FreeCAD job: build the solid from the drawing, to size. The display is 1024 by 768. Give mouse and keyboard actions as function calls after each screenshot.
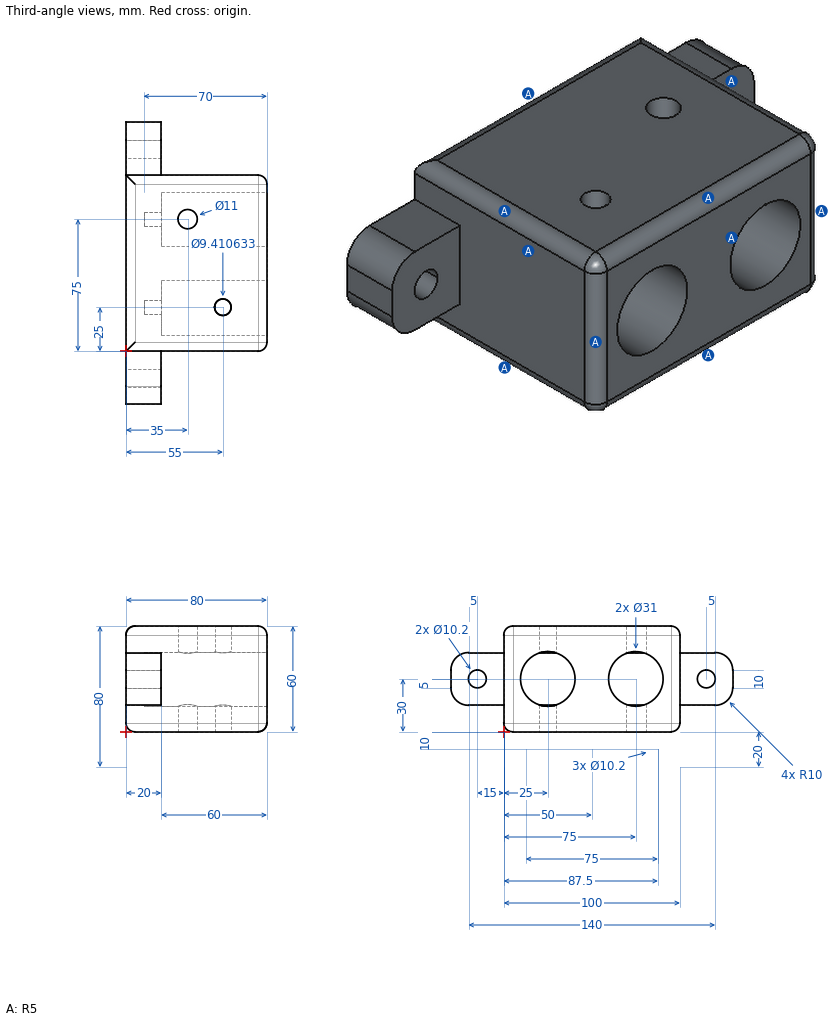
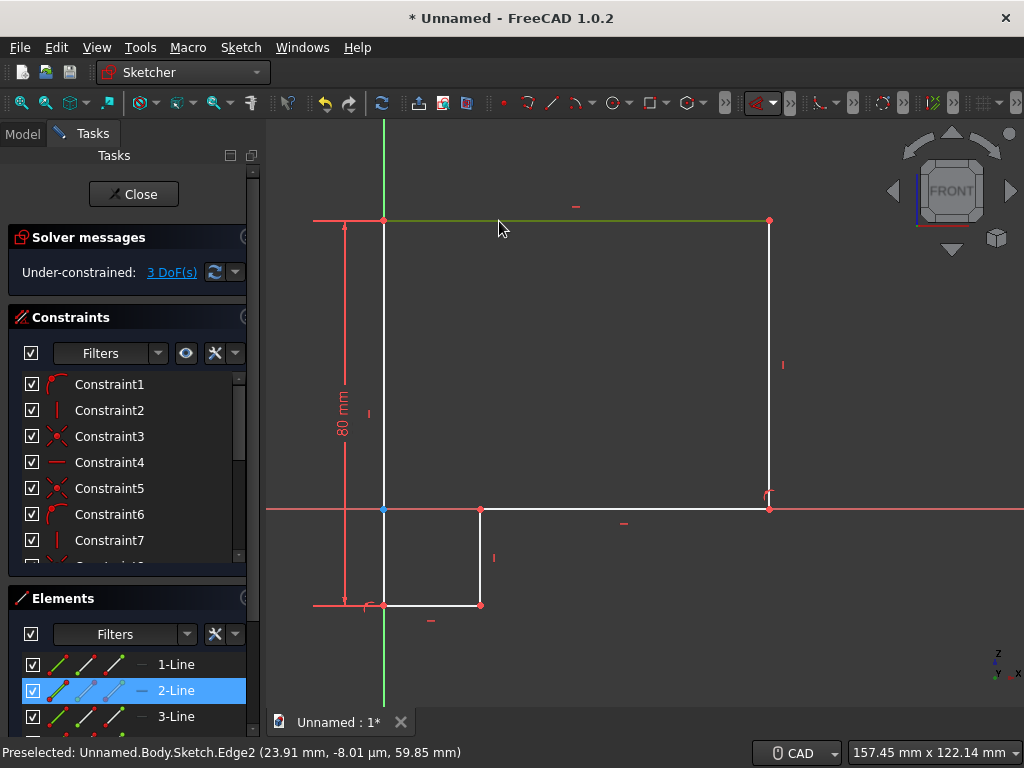
key(l)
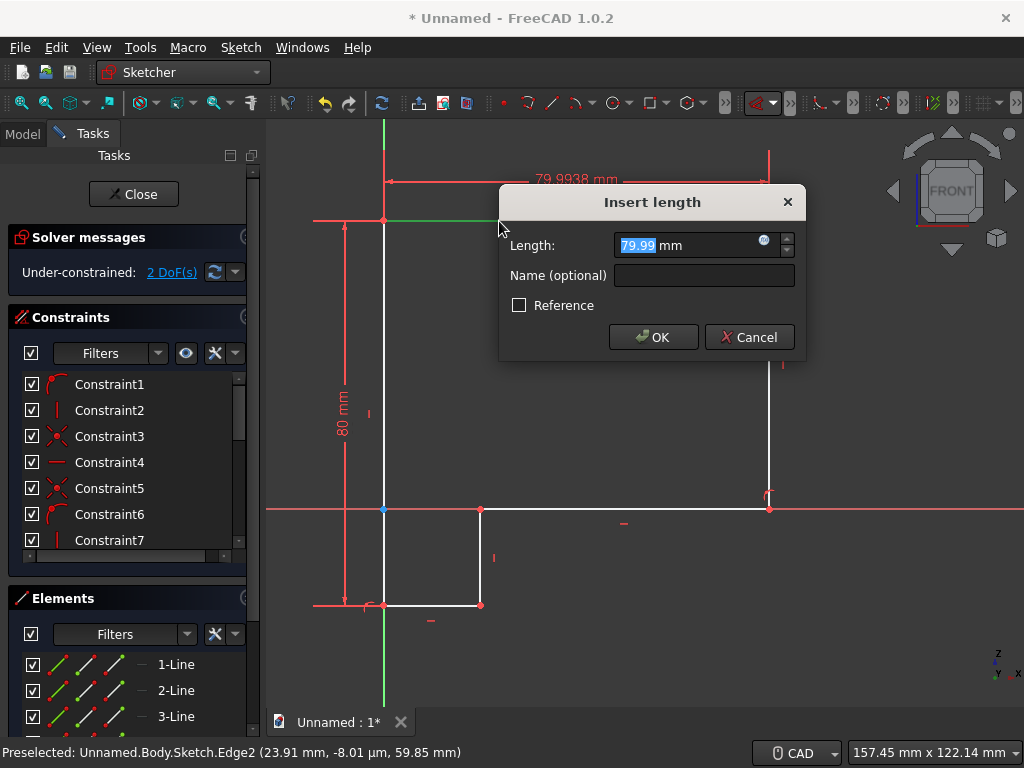
text(80)
key(Return)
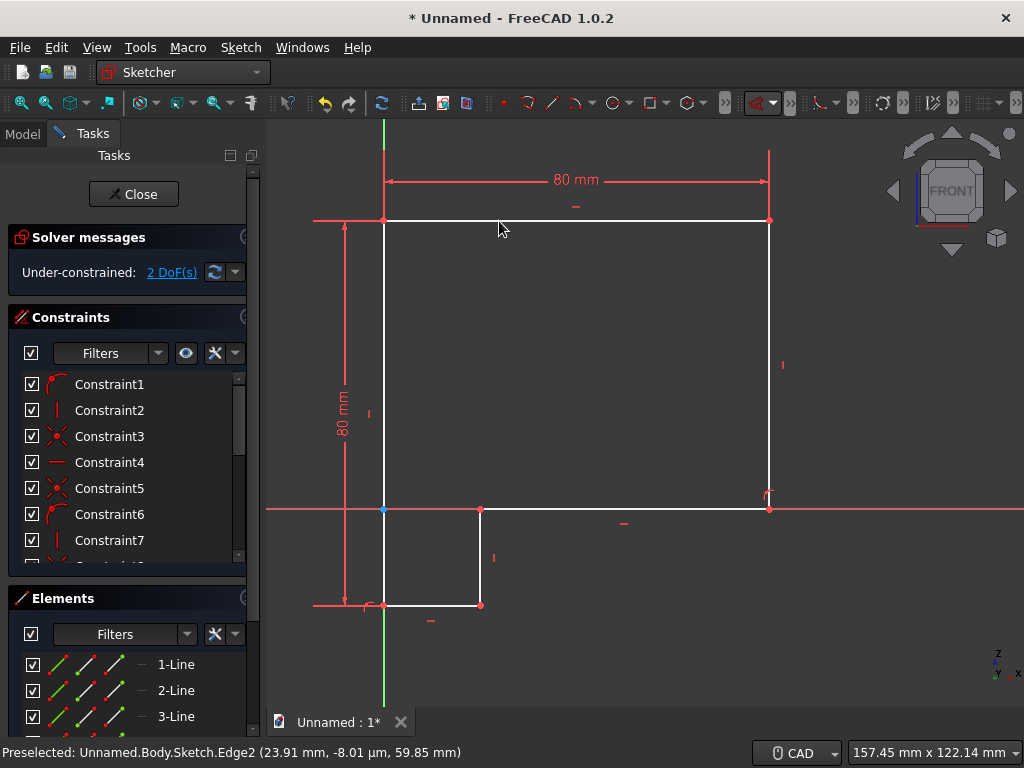
click(769, 307)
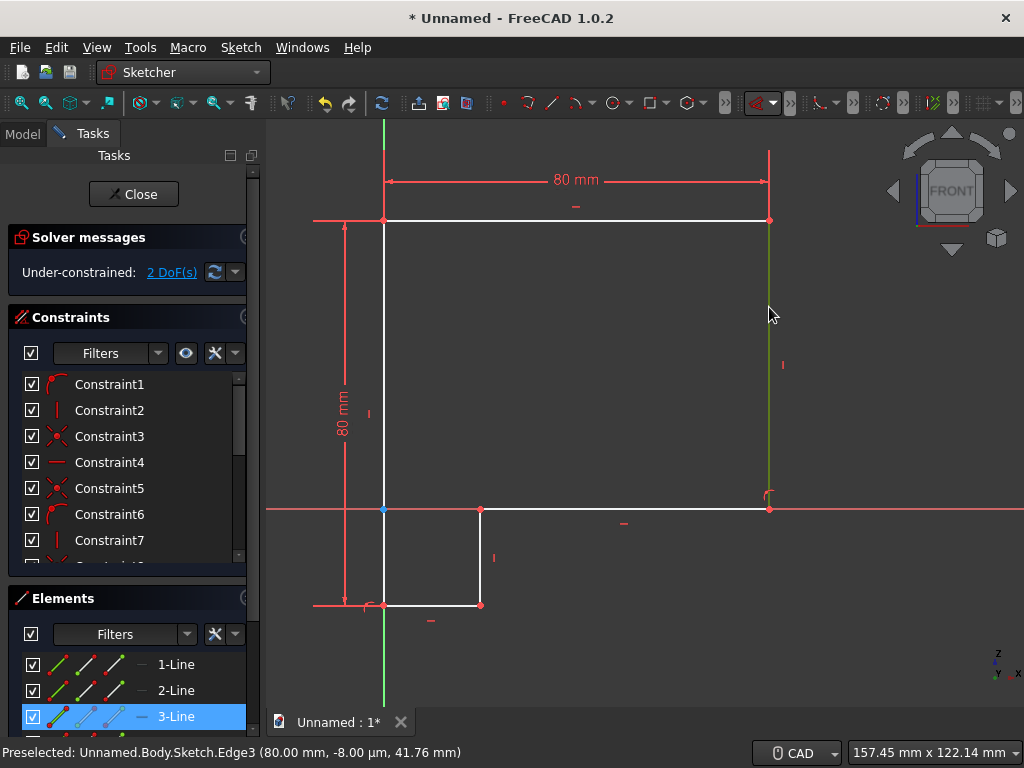
key(i)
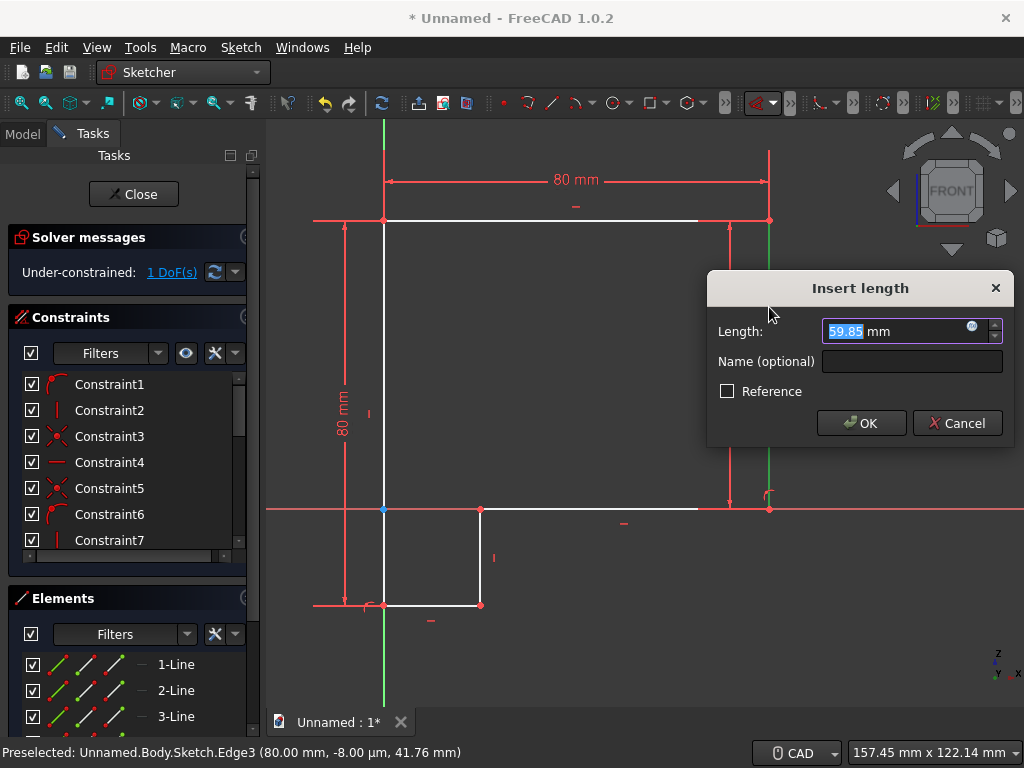
text(60)
key(Return)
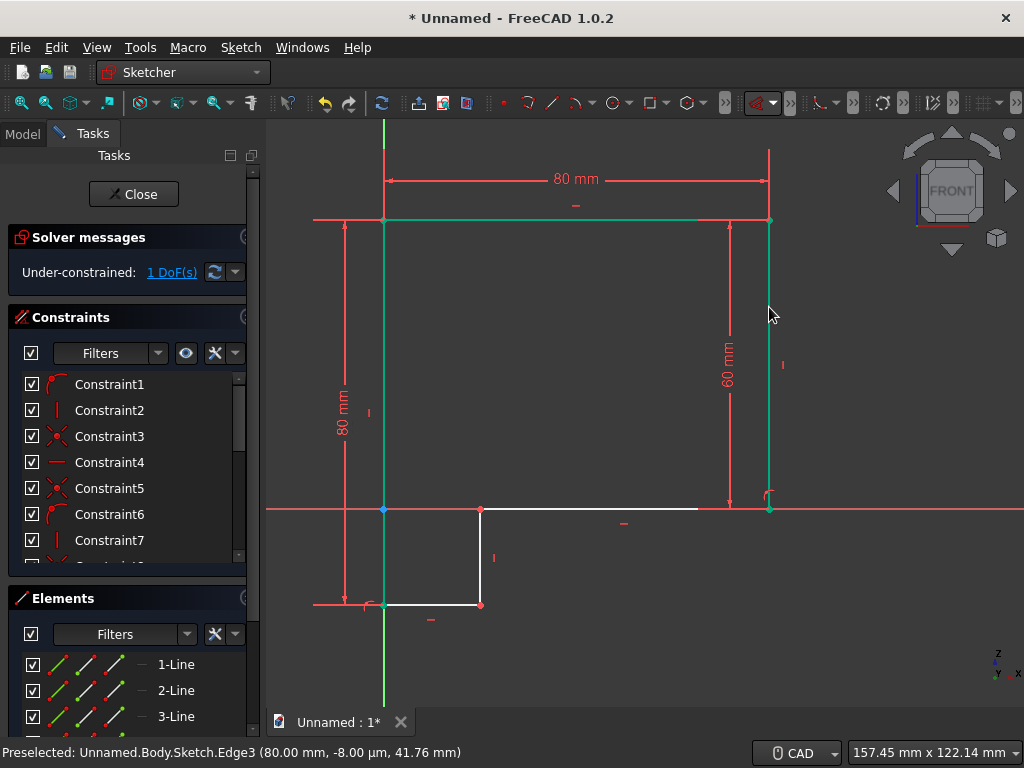
click(682, 509)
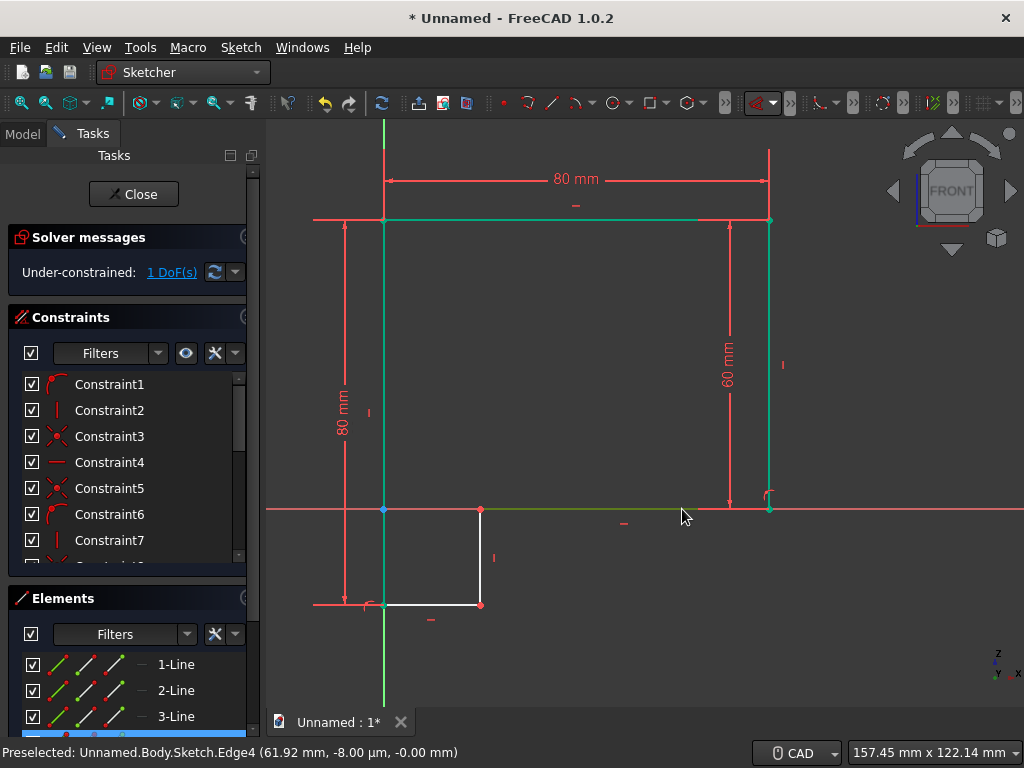
key(l)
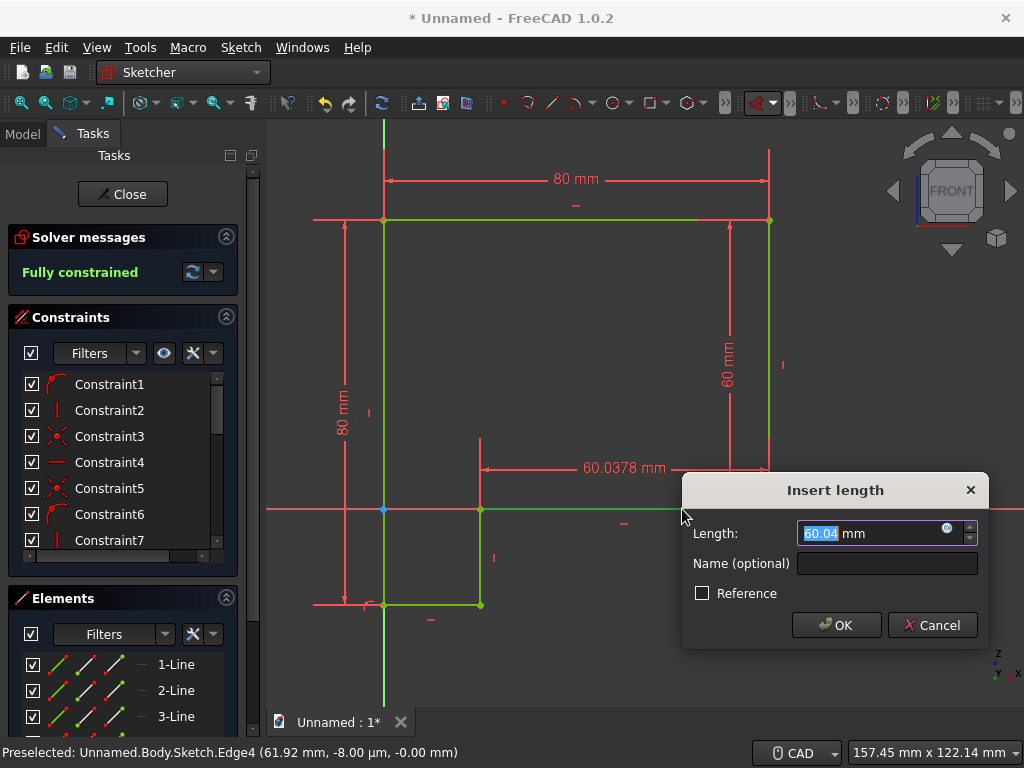
text(60)
key(Return)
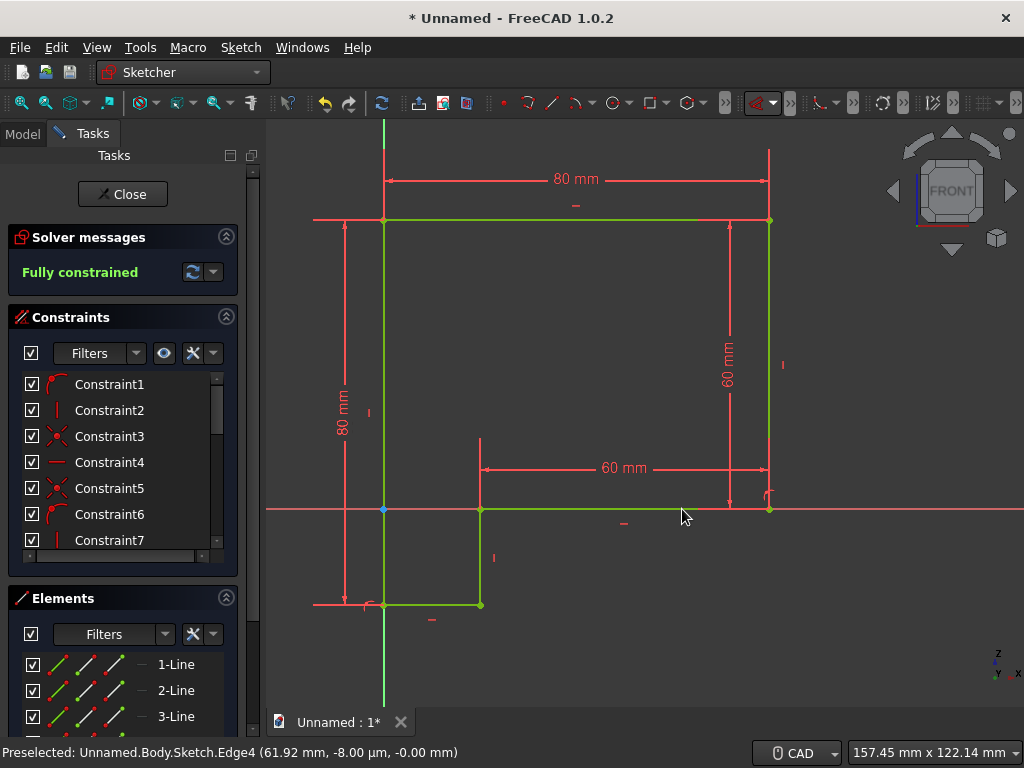
click(123, 194)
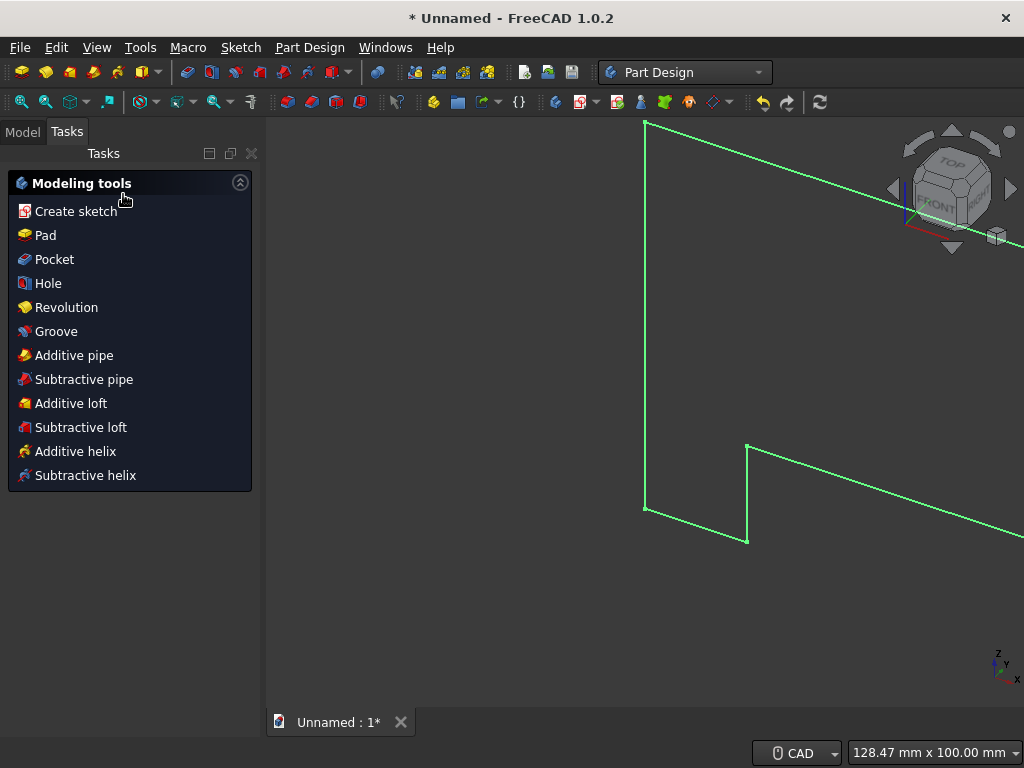
click(22, 72)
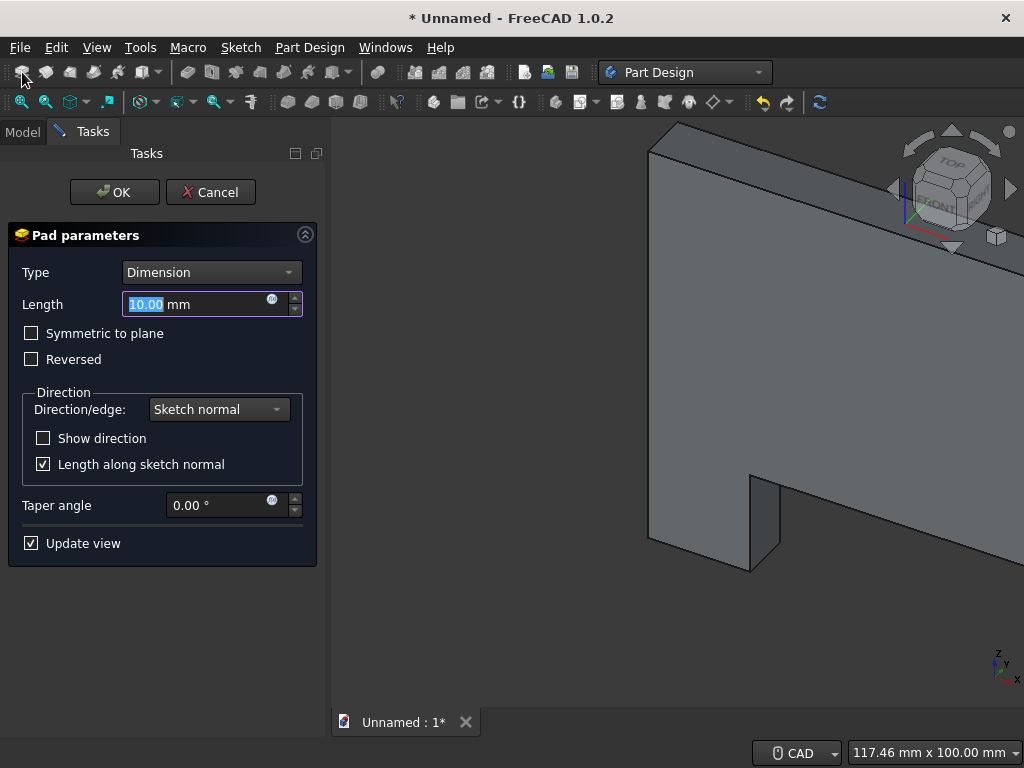
text(100)
key(Tab)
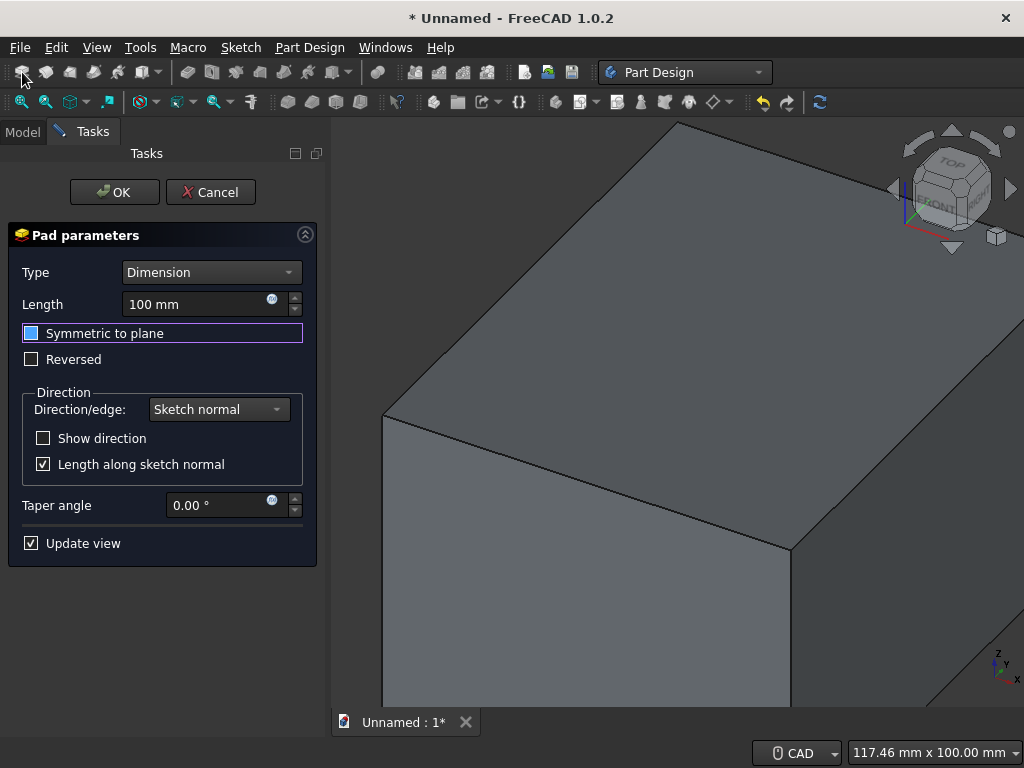
click(30, 359)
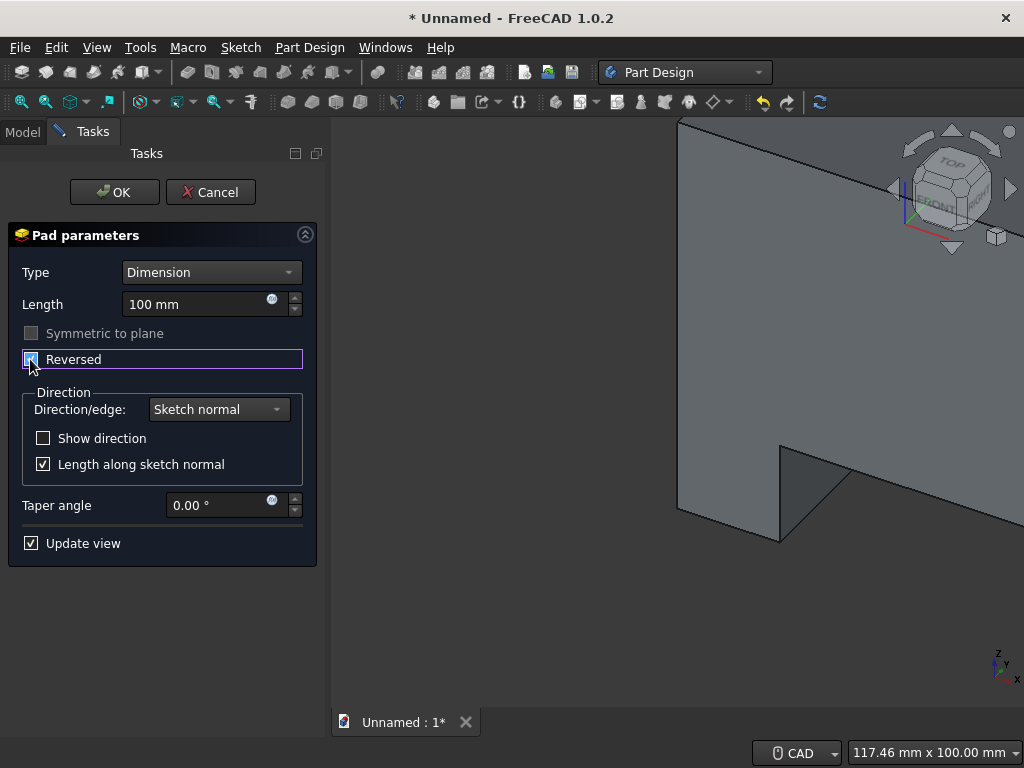
click(115, 192)